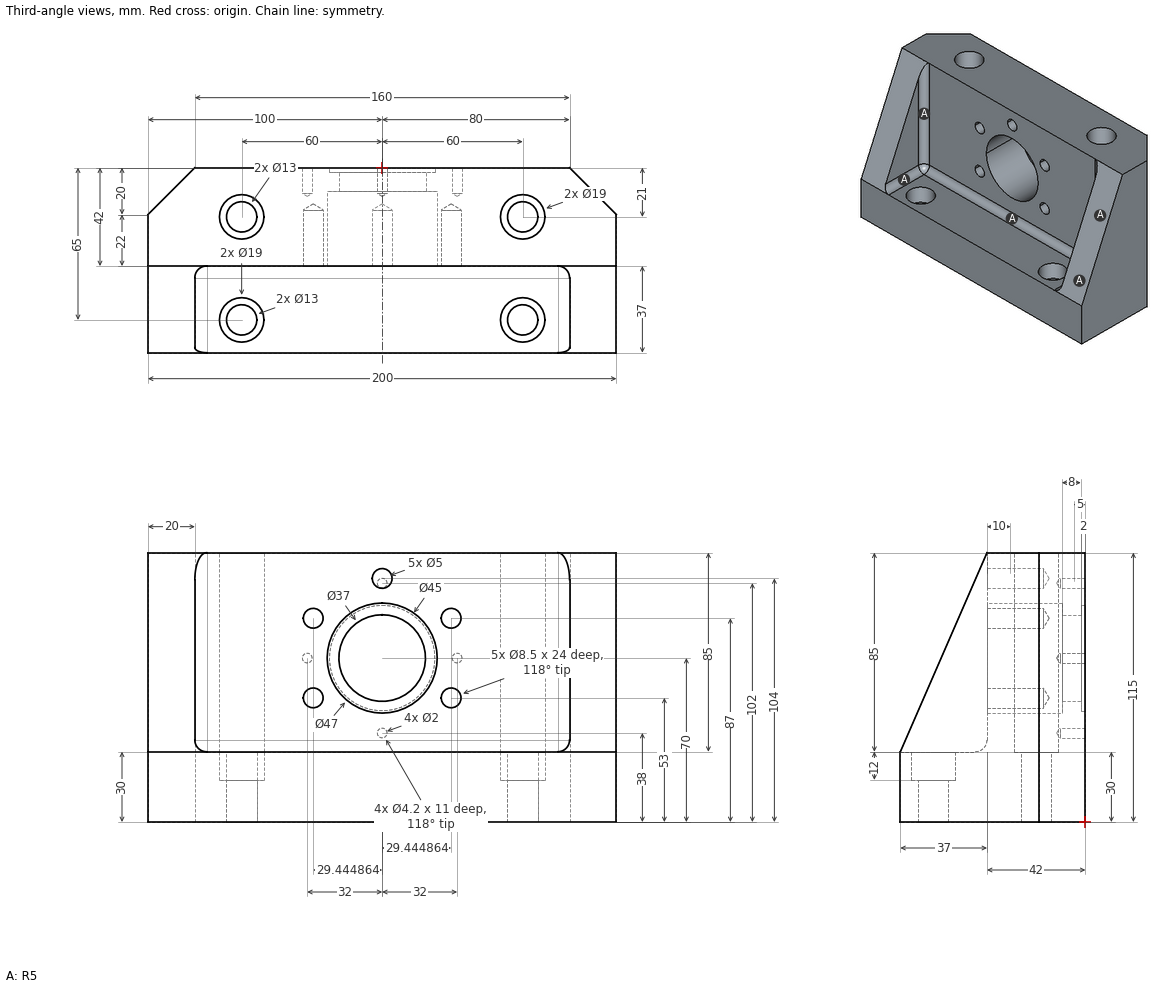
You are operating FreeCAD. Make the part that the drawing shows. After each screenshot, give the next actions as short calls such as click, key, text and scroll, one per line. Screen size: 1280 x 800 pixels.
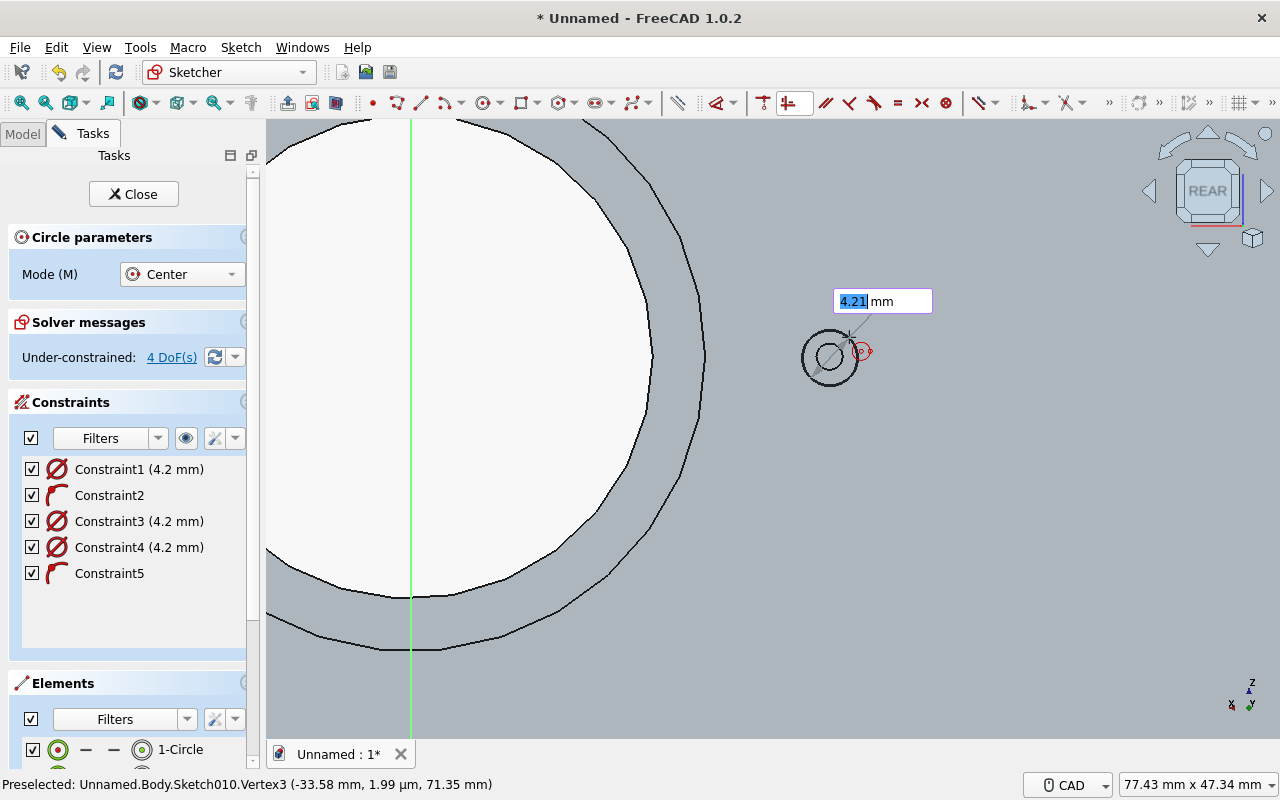
text(4.2)
key(Return)
key(Escape)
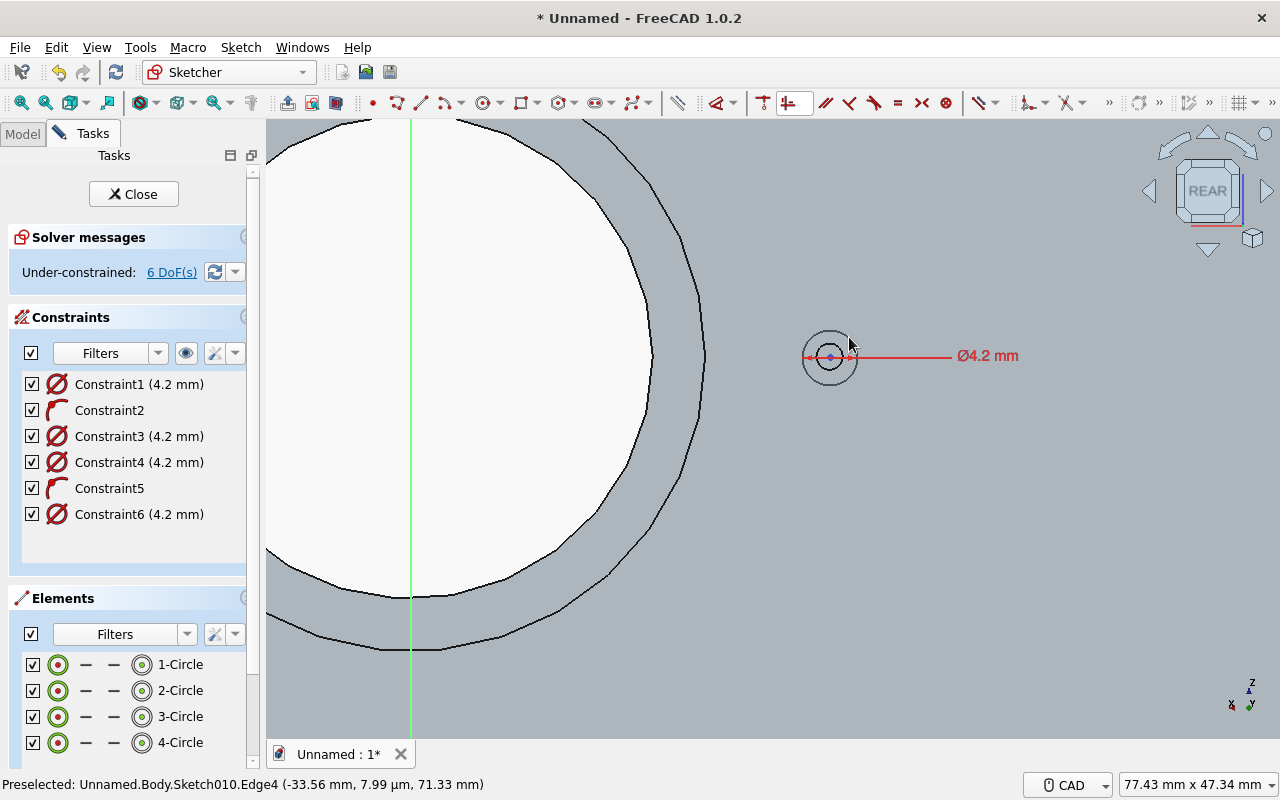
scroll(831, 359, down, 6)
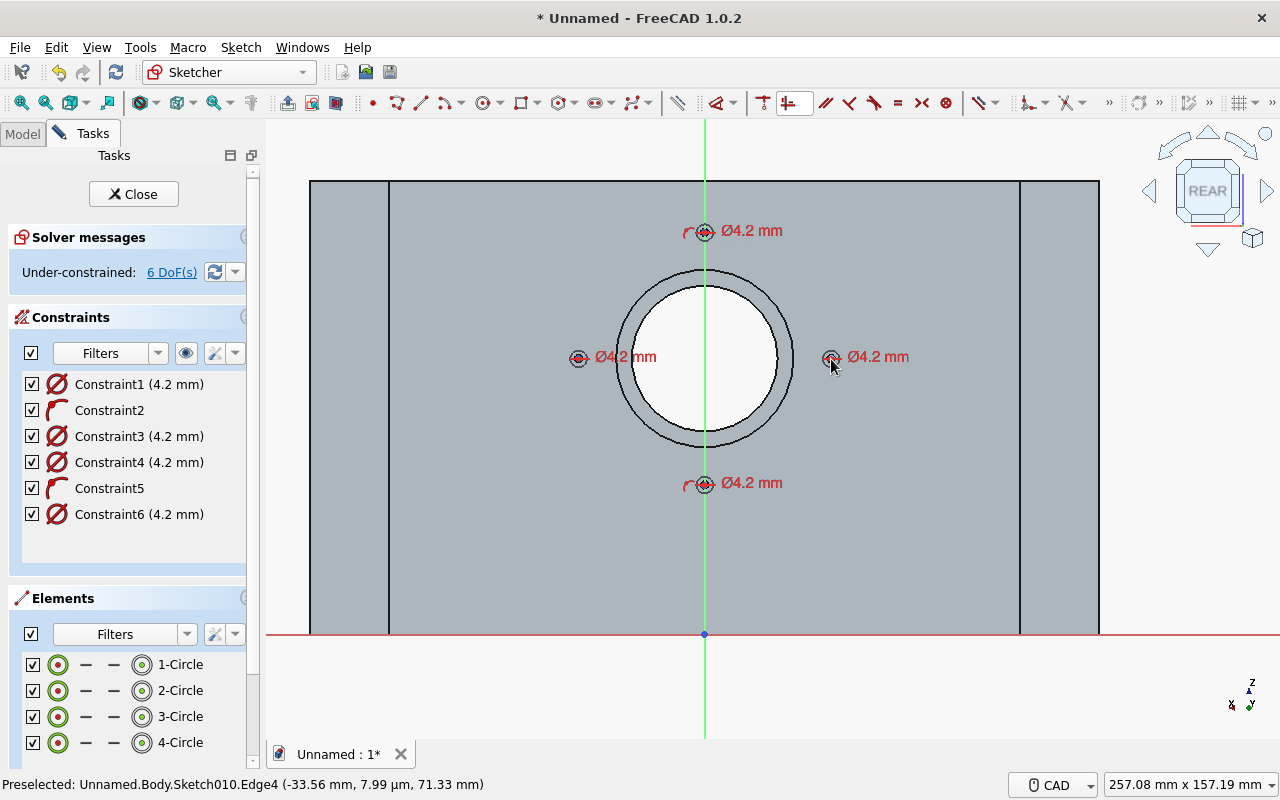
click(579, 359)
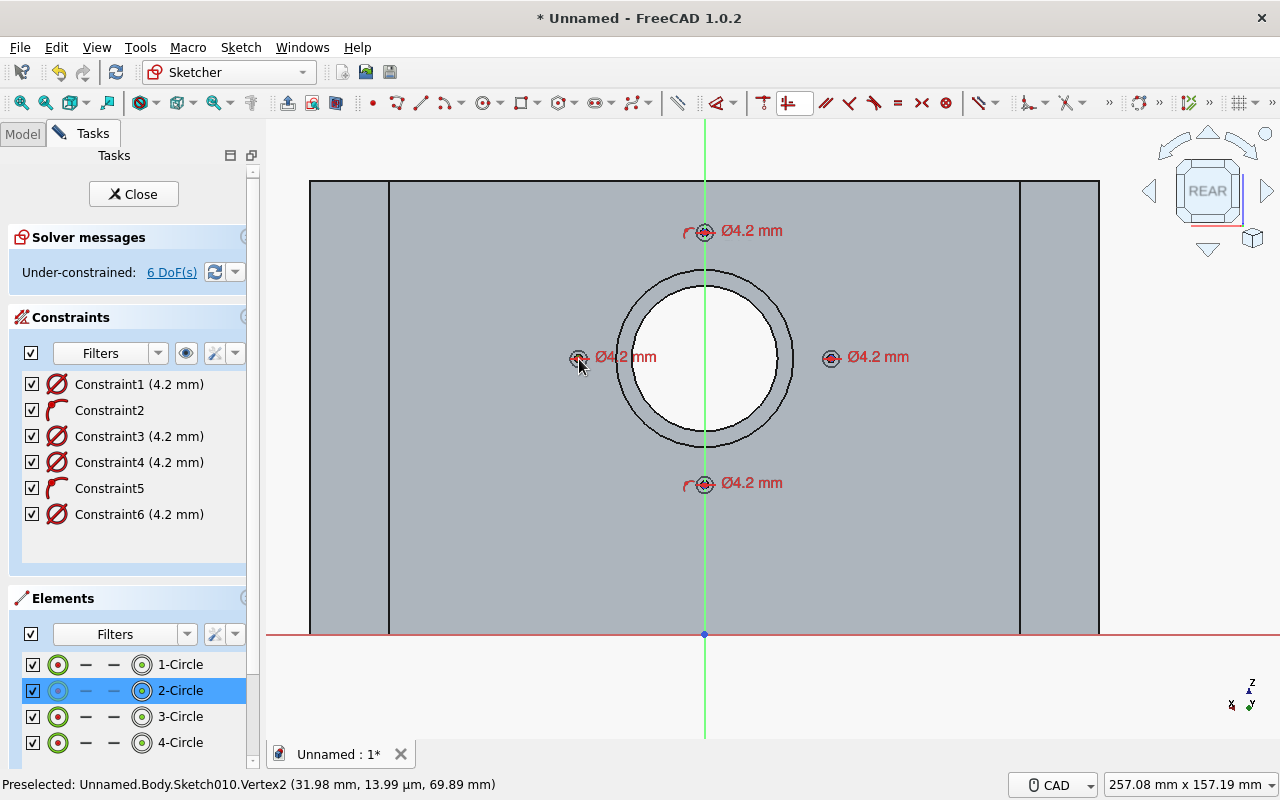
click(831, 359)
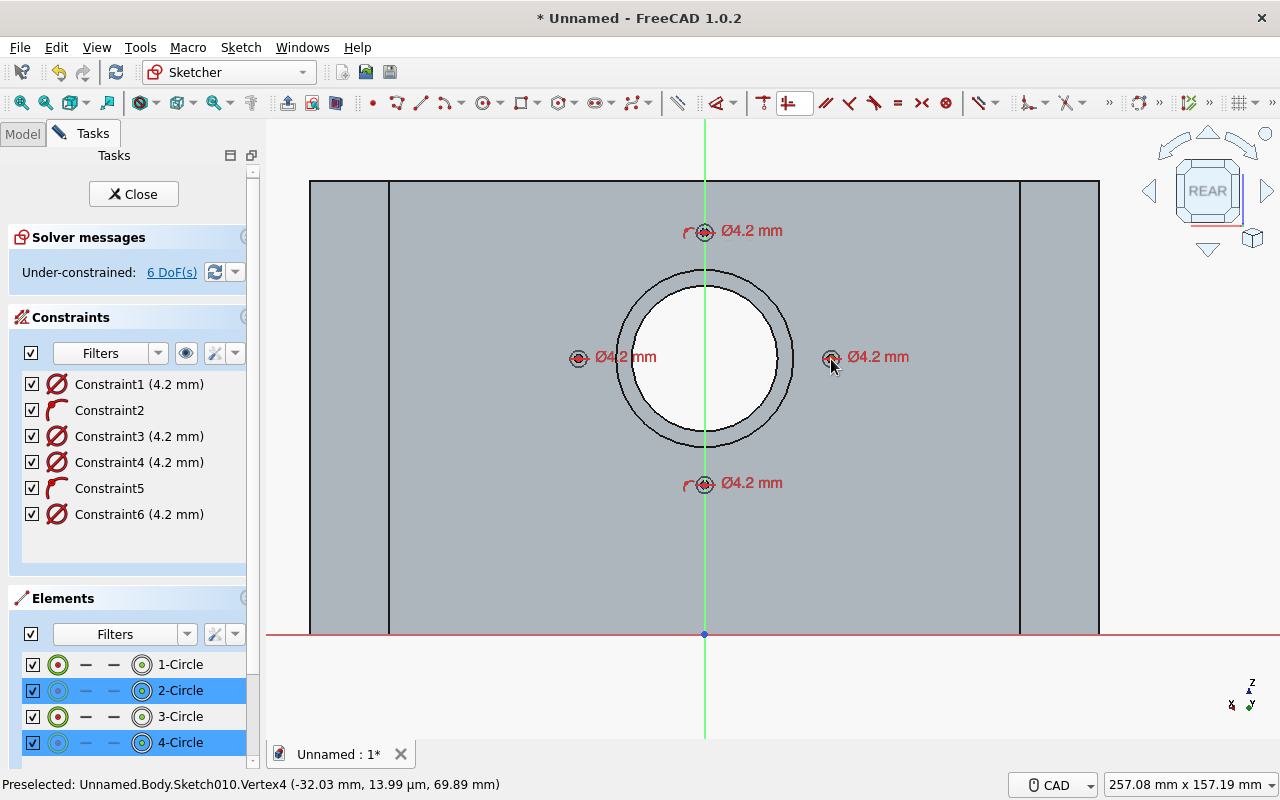
click(808, 104)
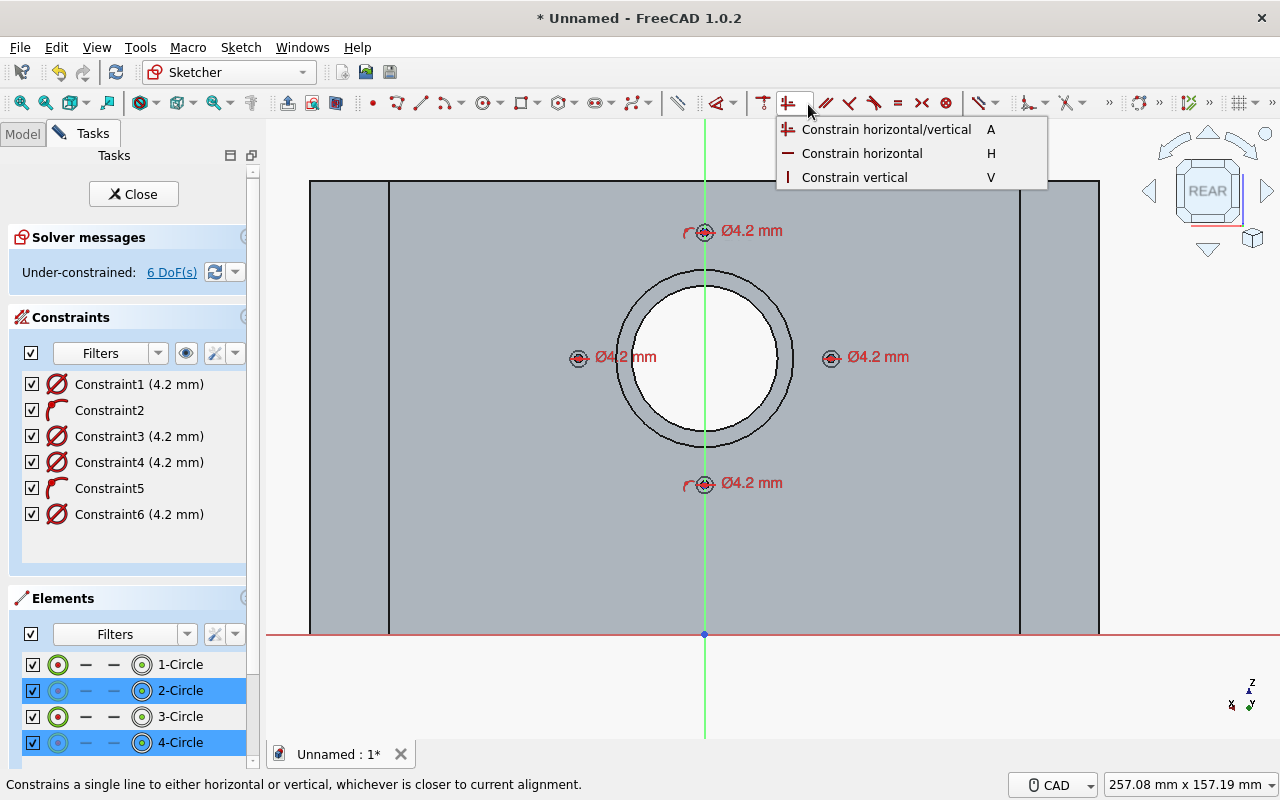
click(912, 153)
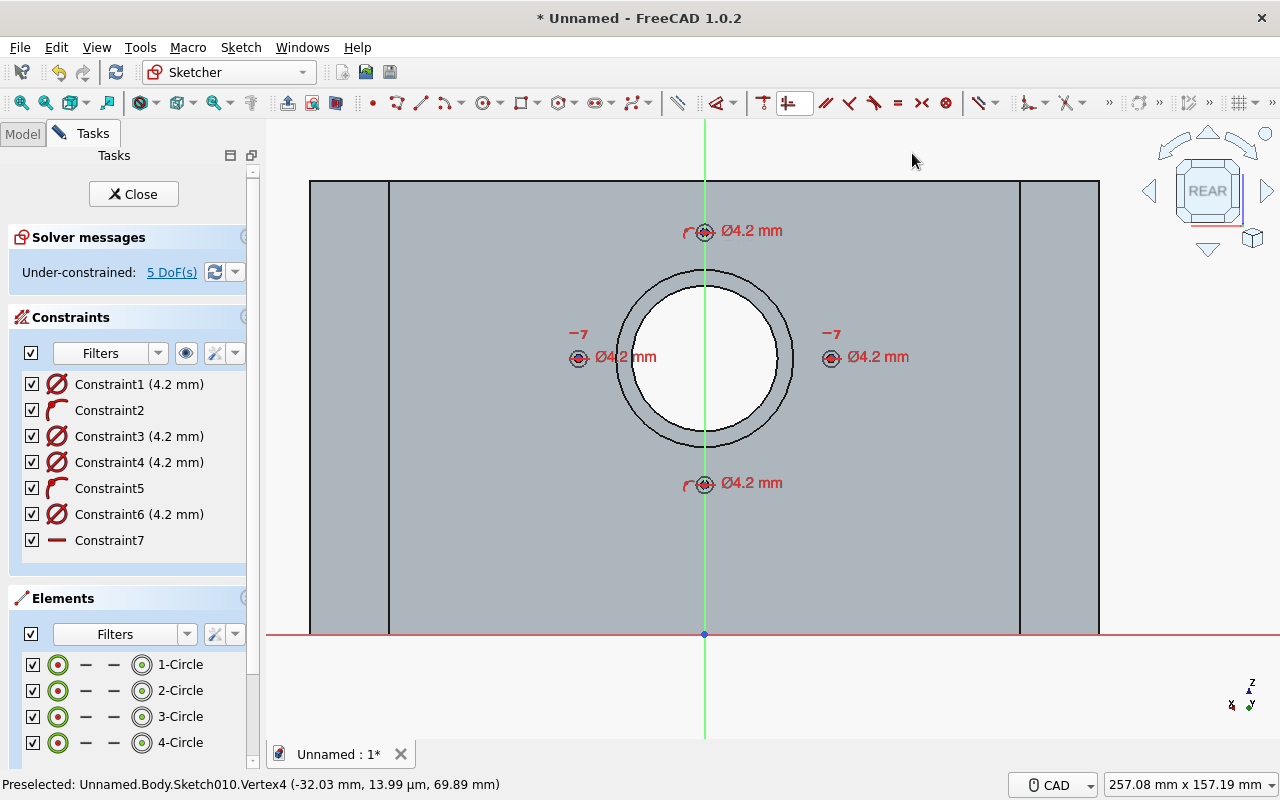
click(716, 104)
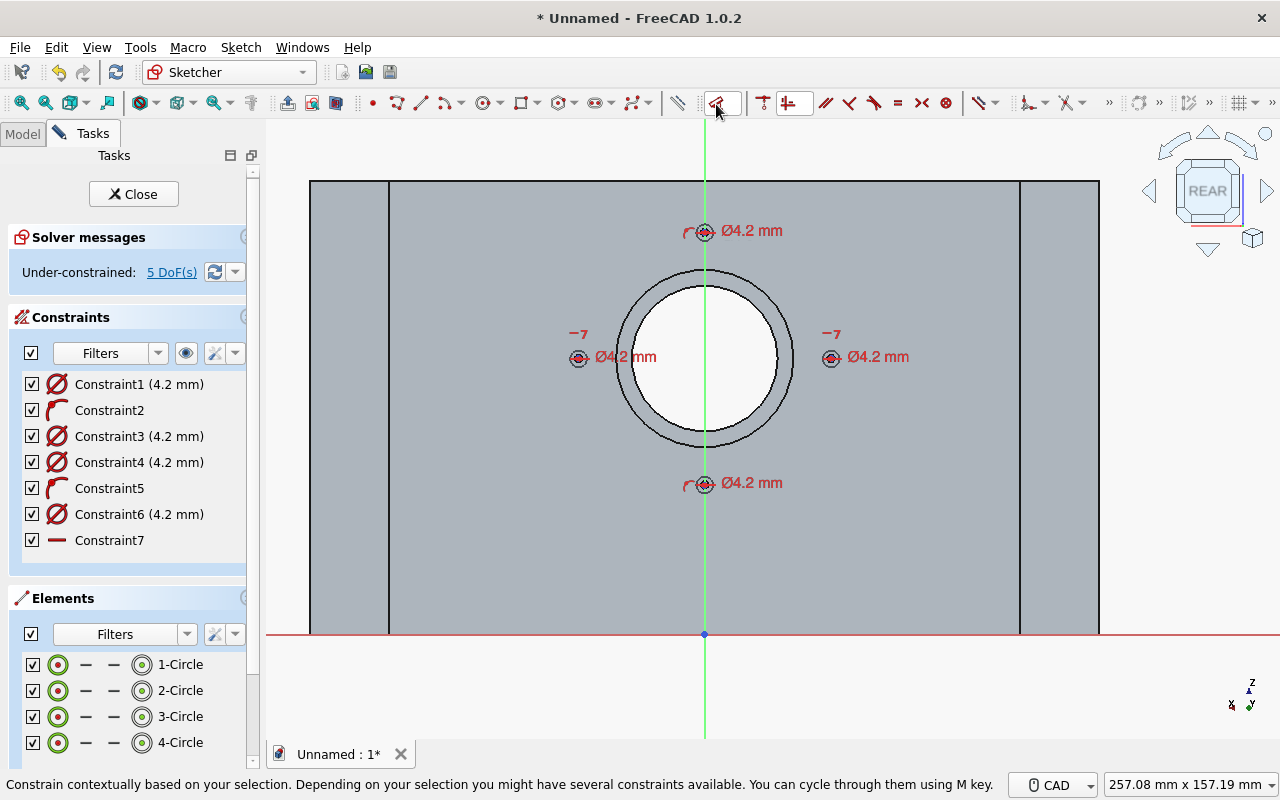
click(705, 485)
click(739, 560)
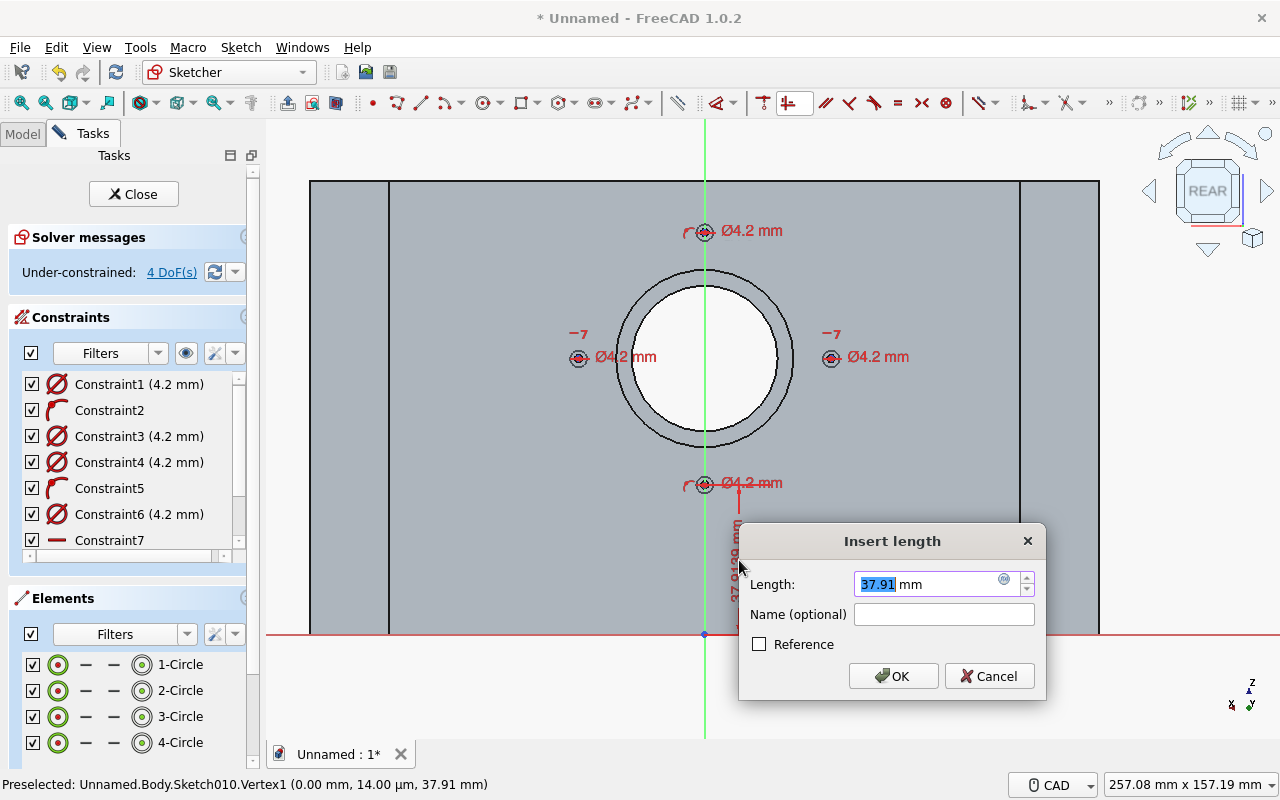
text(38)
key(Return)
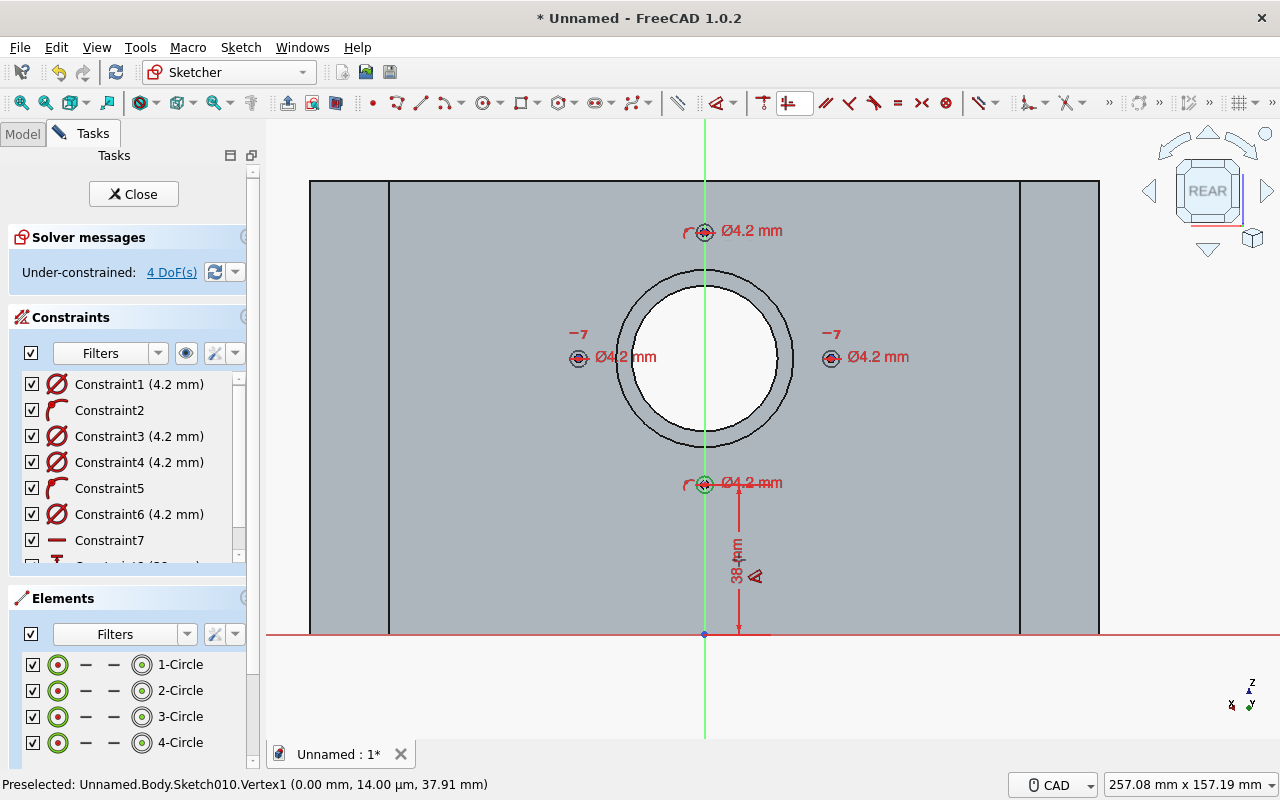
click(579, 359)
click(642, 669)